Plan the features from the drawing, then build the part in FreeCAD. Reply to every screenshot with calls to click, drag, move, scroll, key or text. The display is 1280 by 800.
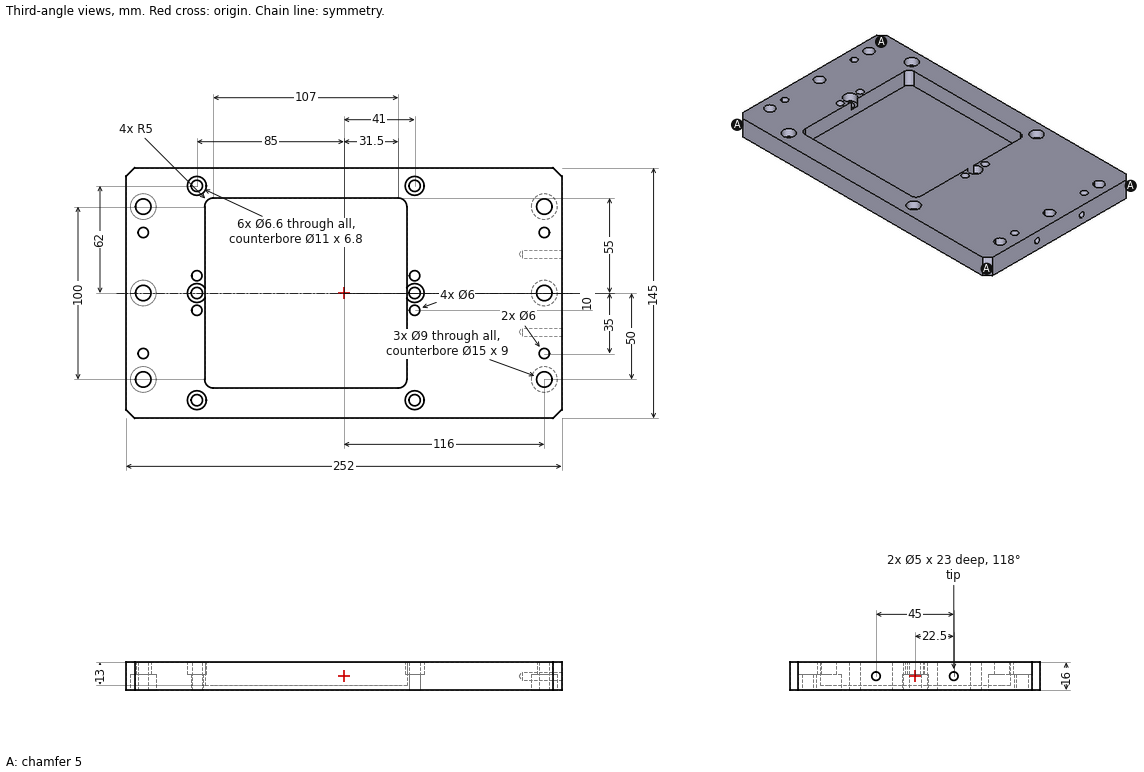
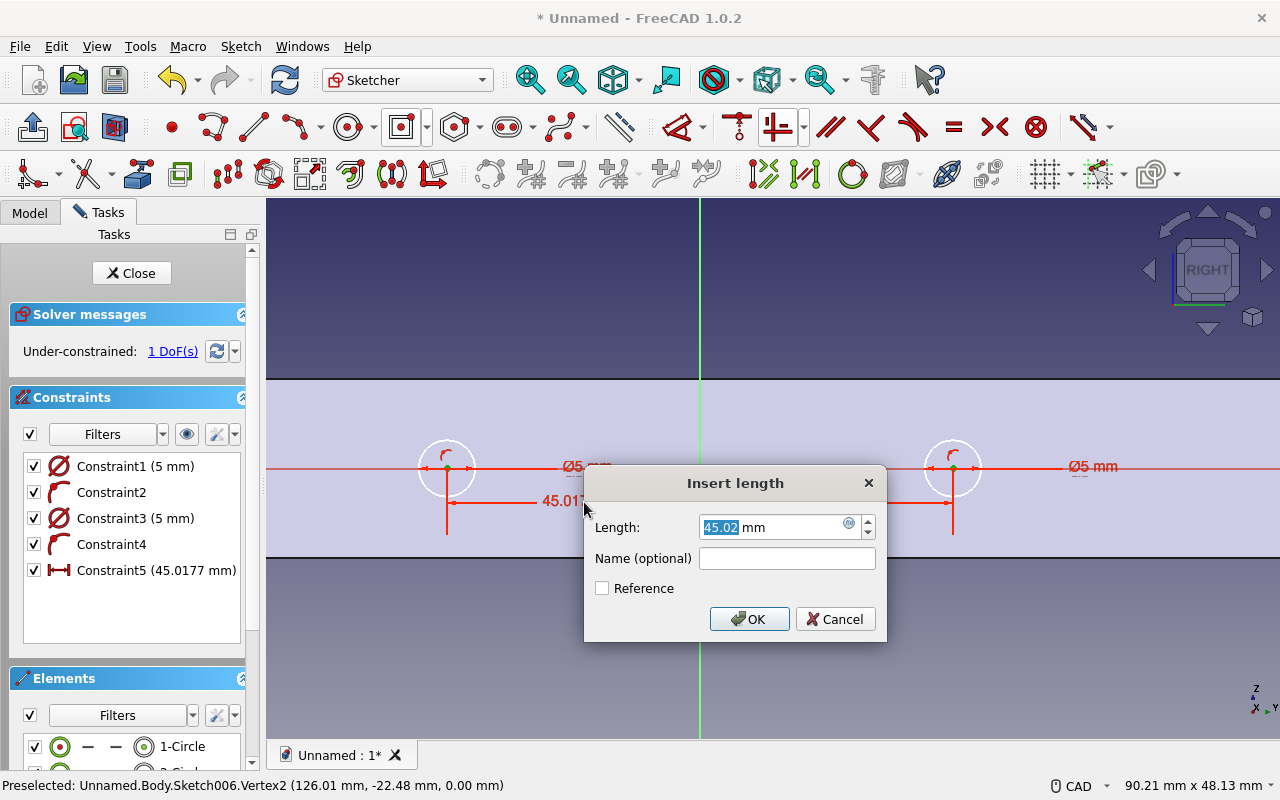
text(45)
key(Return)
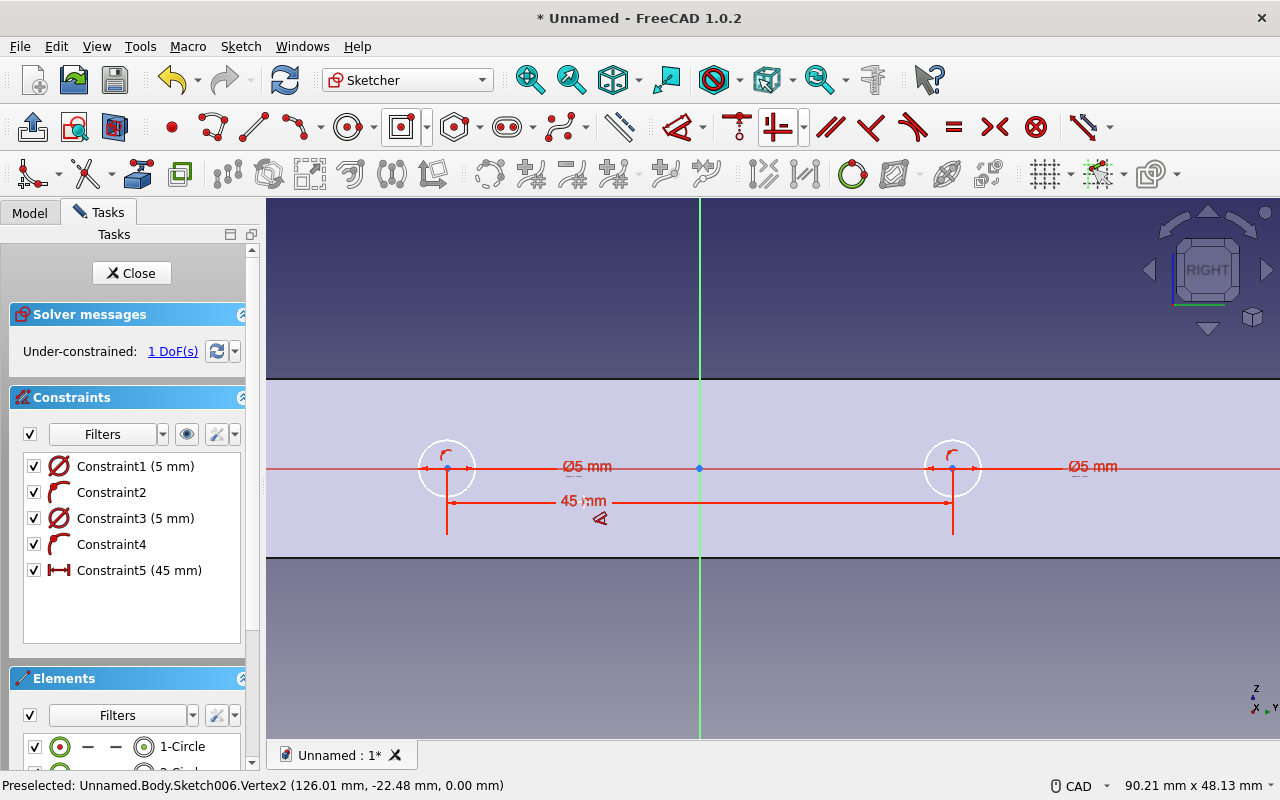
click(953, 468)
click(826, 502)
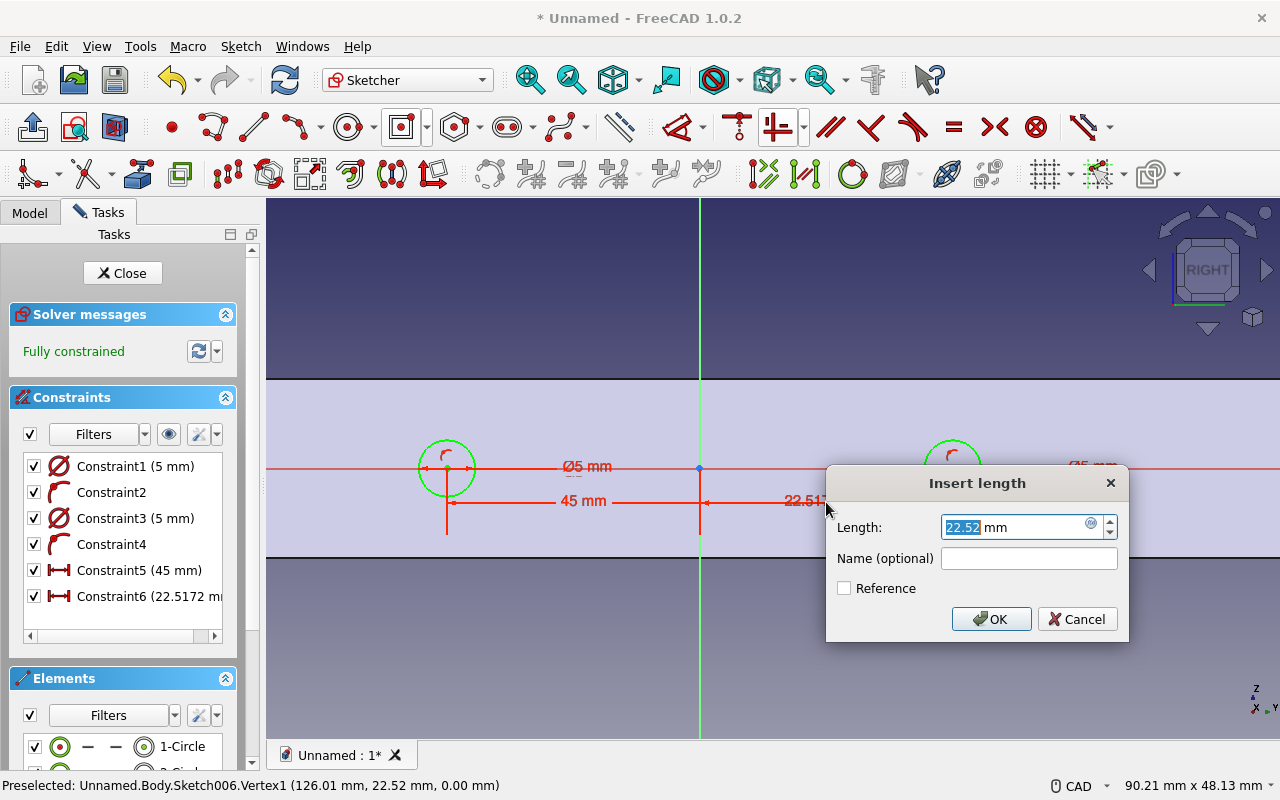
text(22.5)
key(Return)
key(Escape)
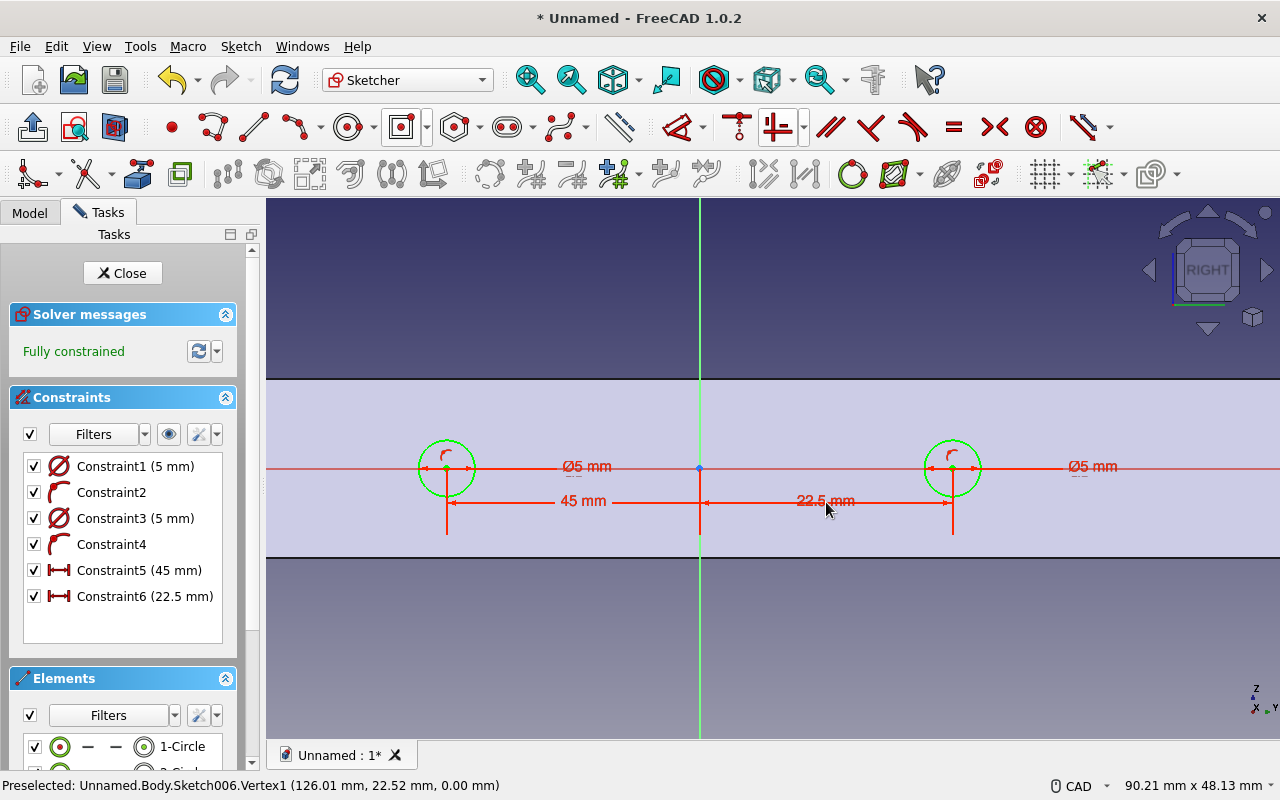
click(123, 273)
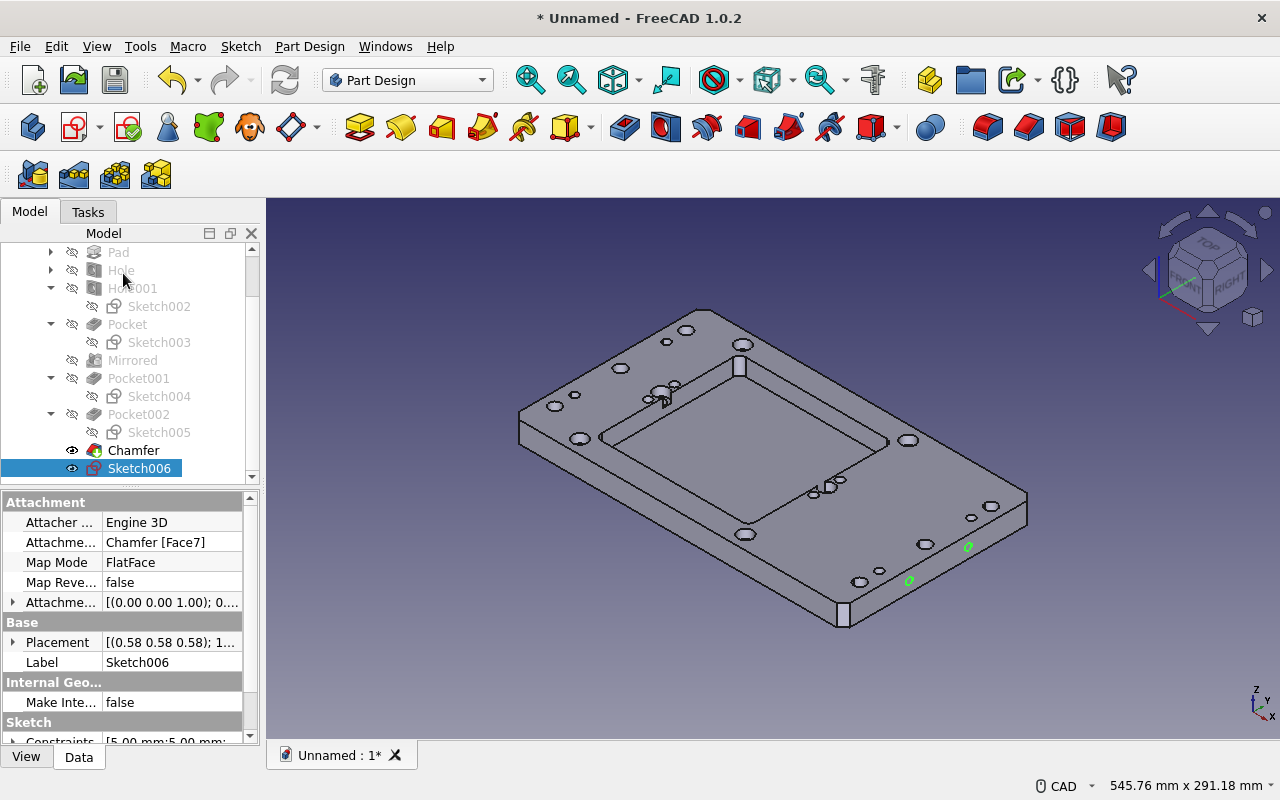
click(666, 128)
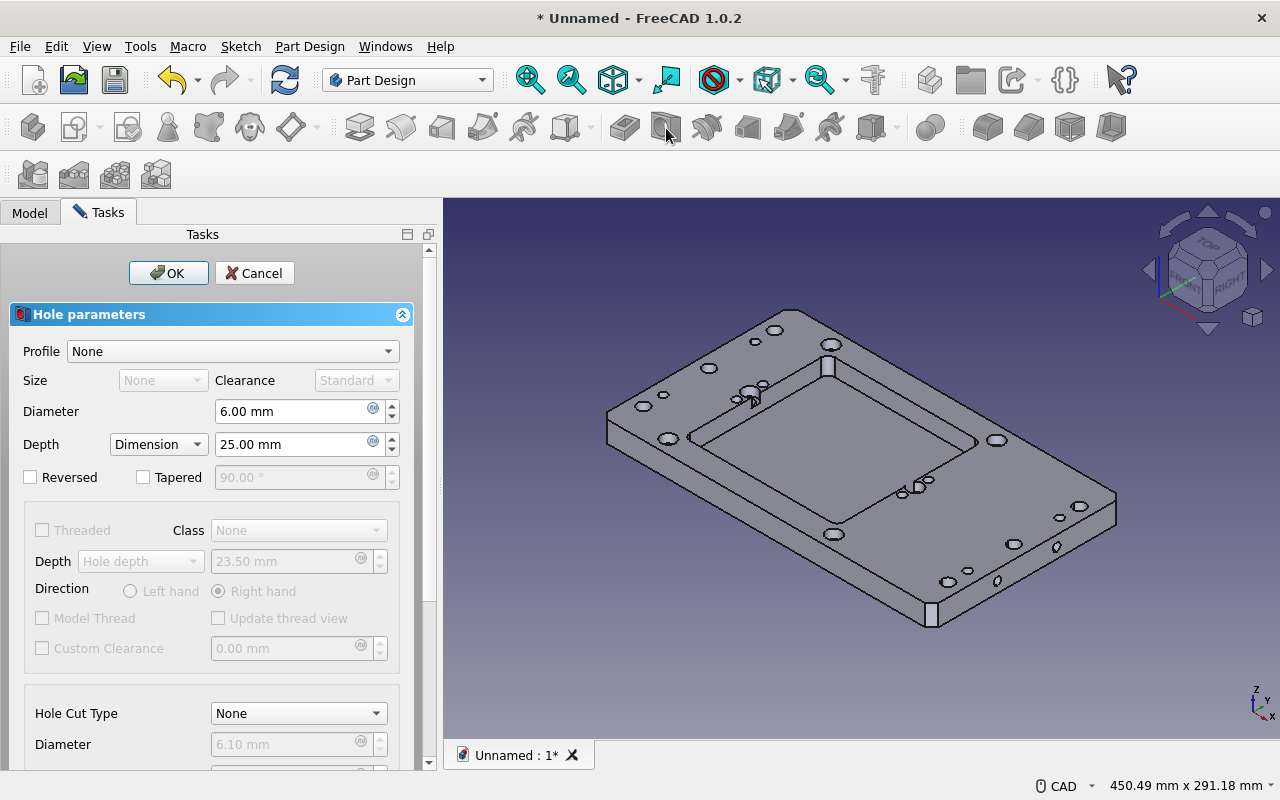
triple_click(300, 412)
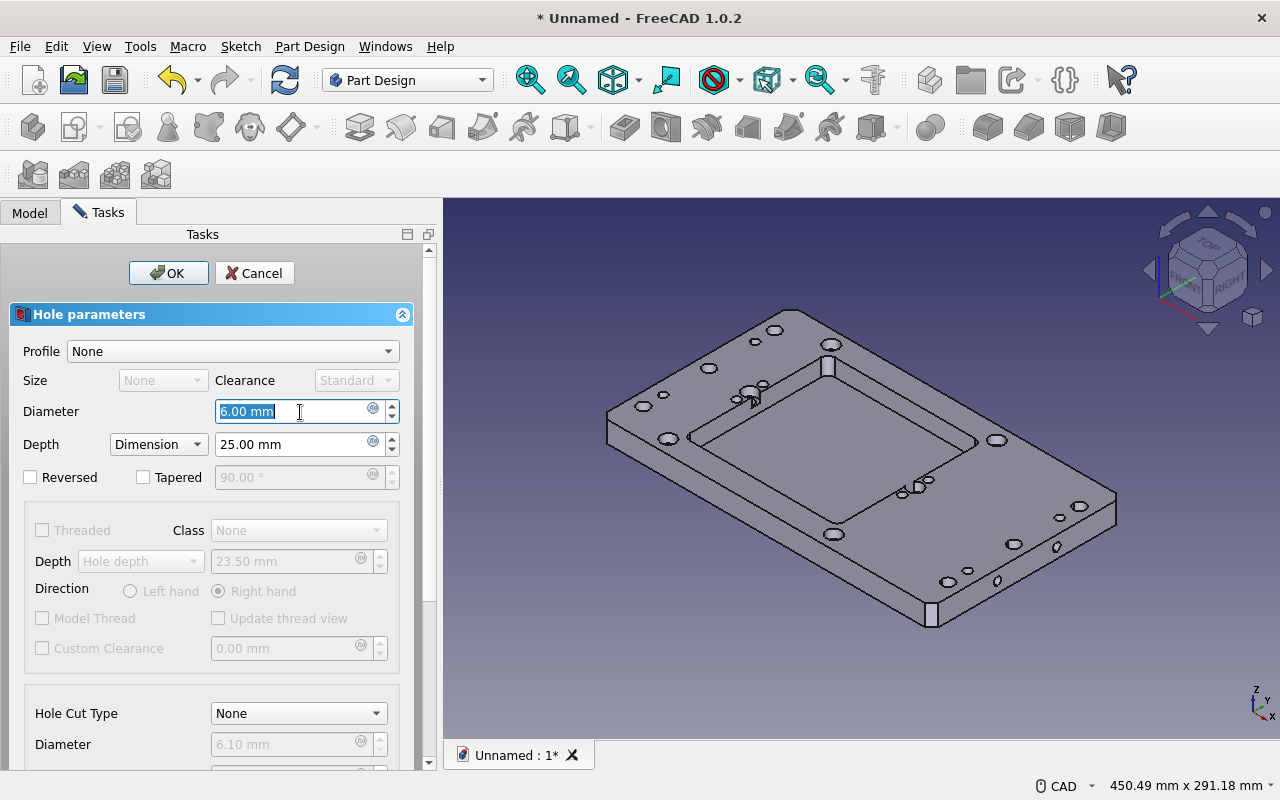
text(5)
key(Tab)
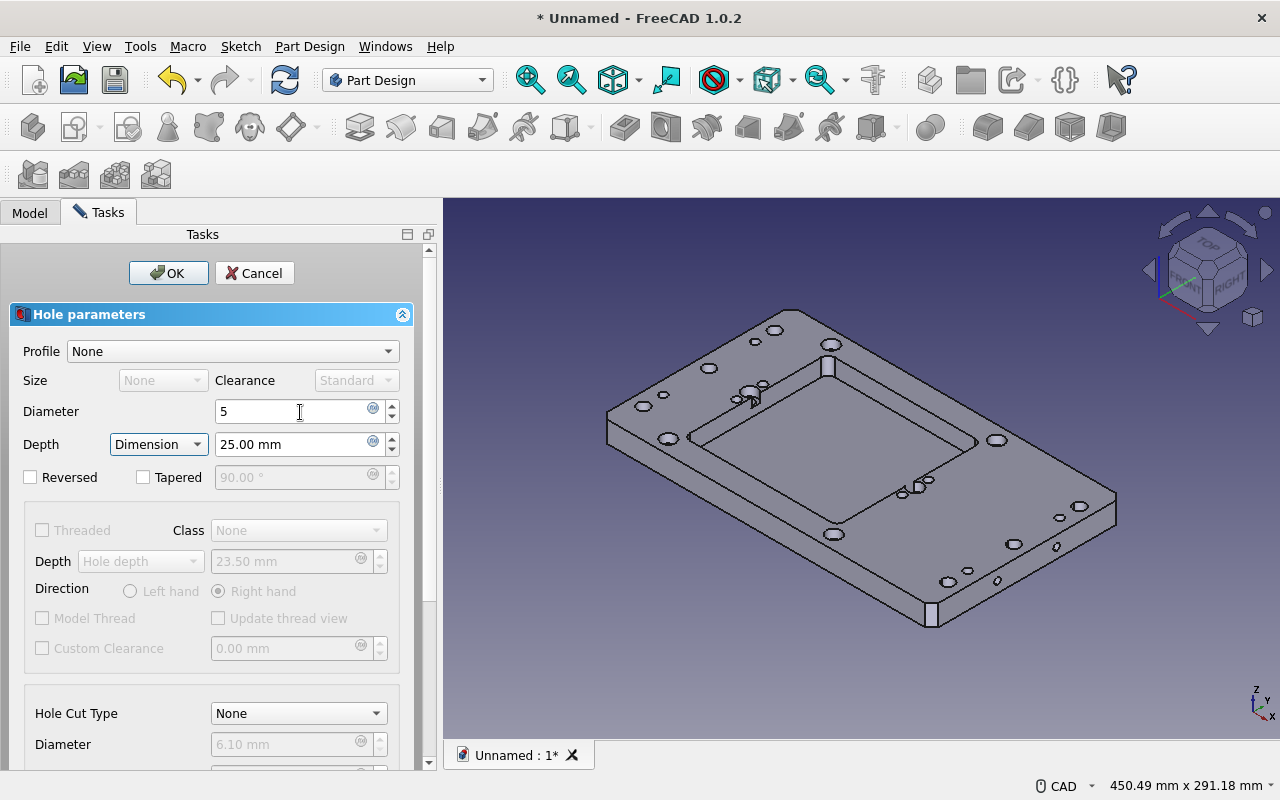
triple_click(300, 444)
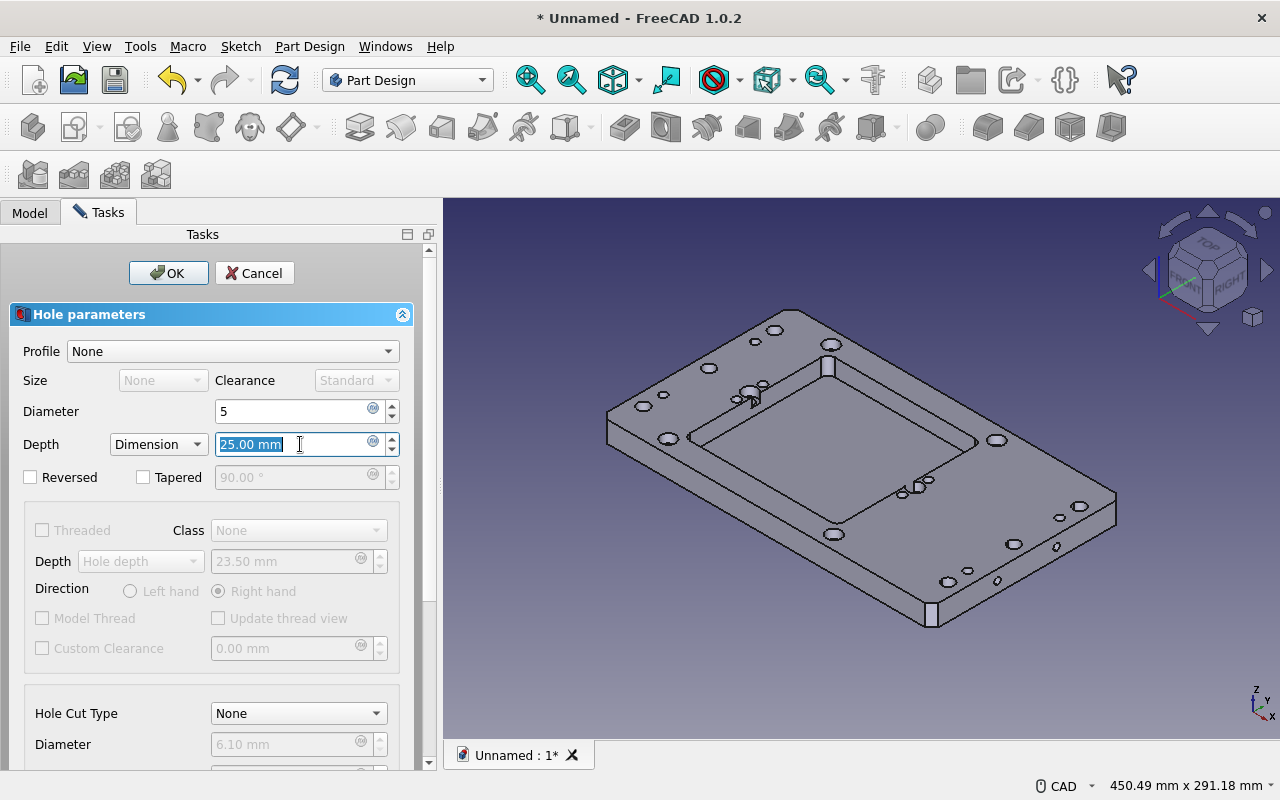
text(23)
key(Tab)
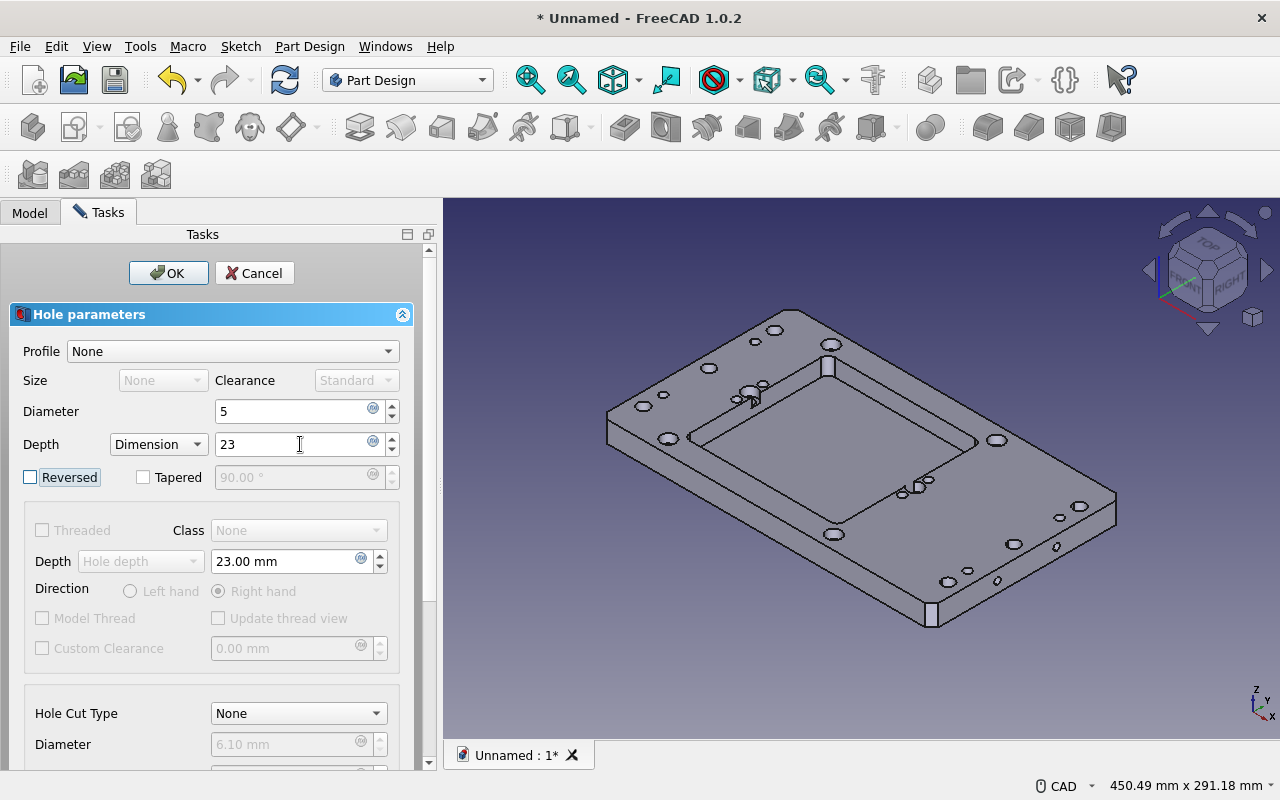
click(169, 273)